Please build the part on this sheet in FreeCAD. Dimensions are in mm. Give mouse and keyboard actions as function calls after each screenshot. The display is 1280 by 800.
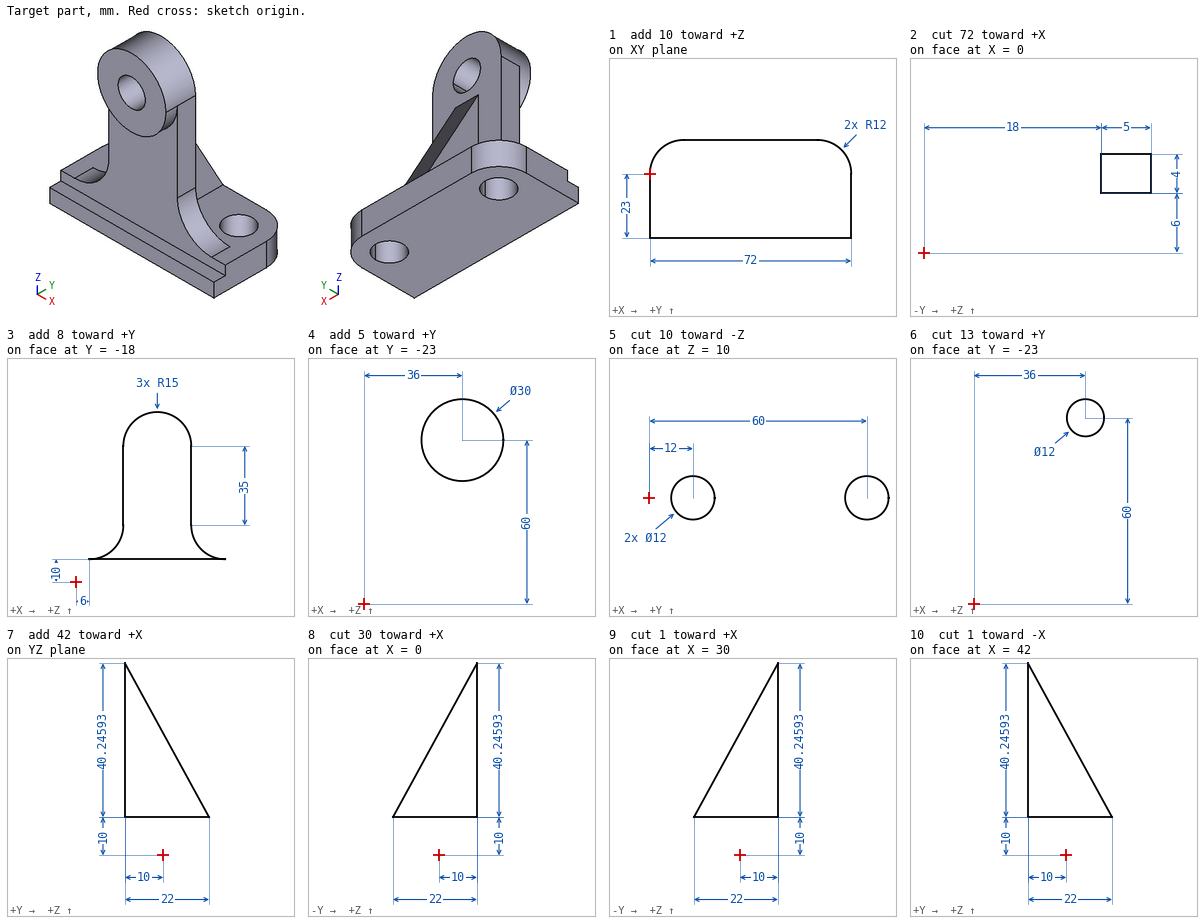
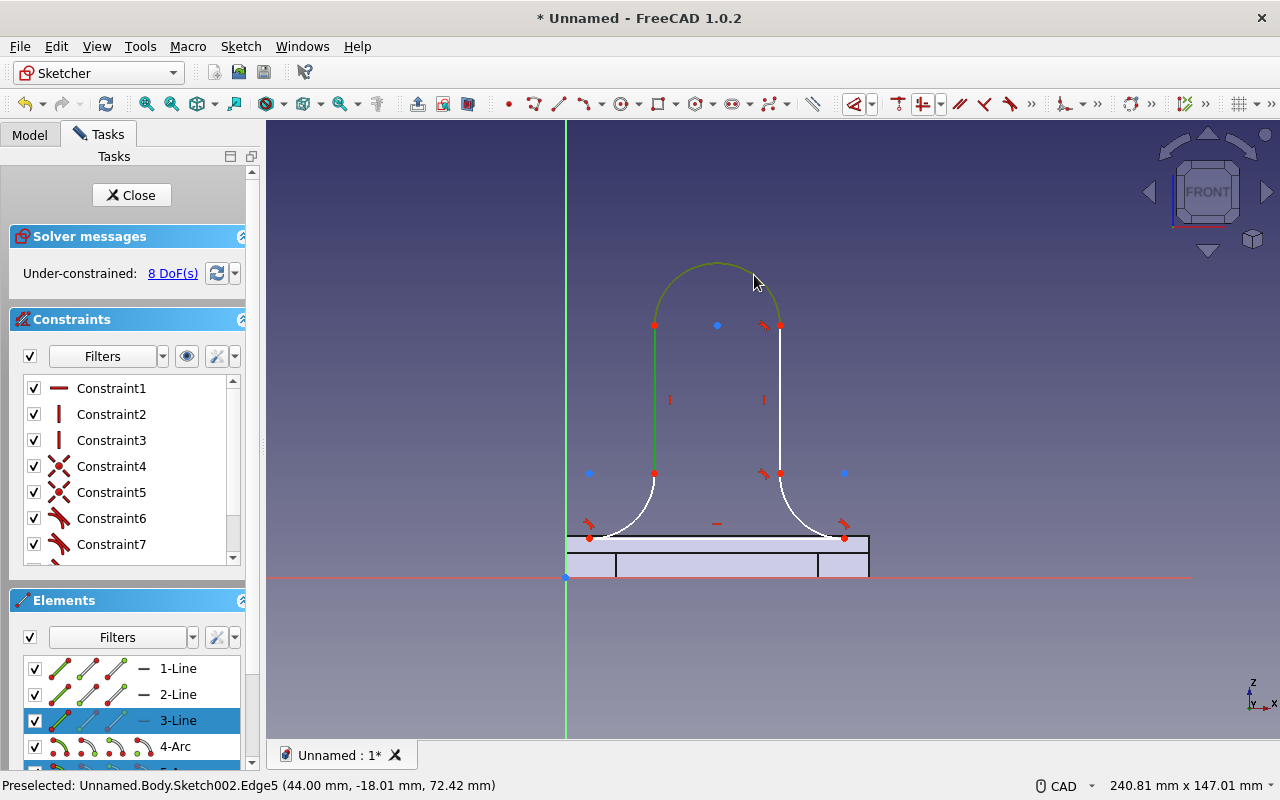
click(1010, 104)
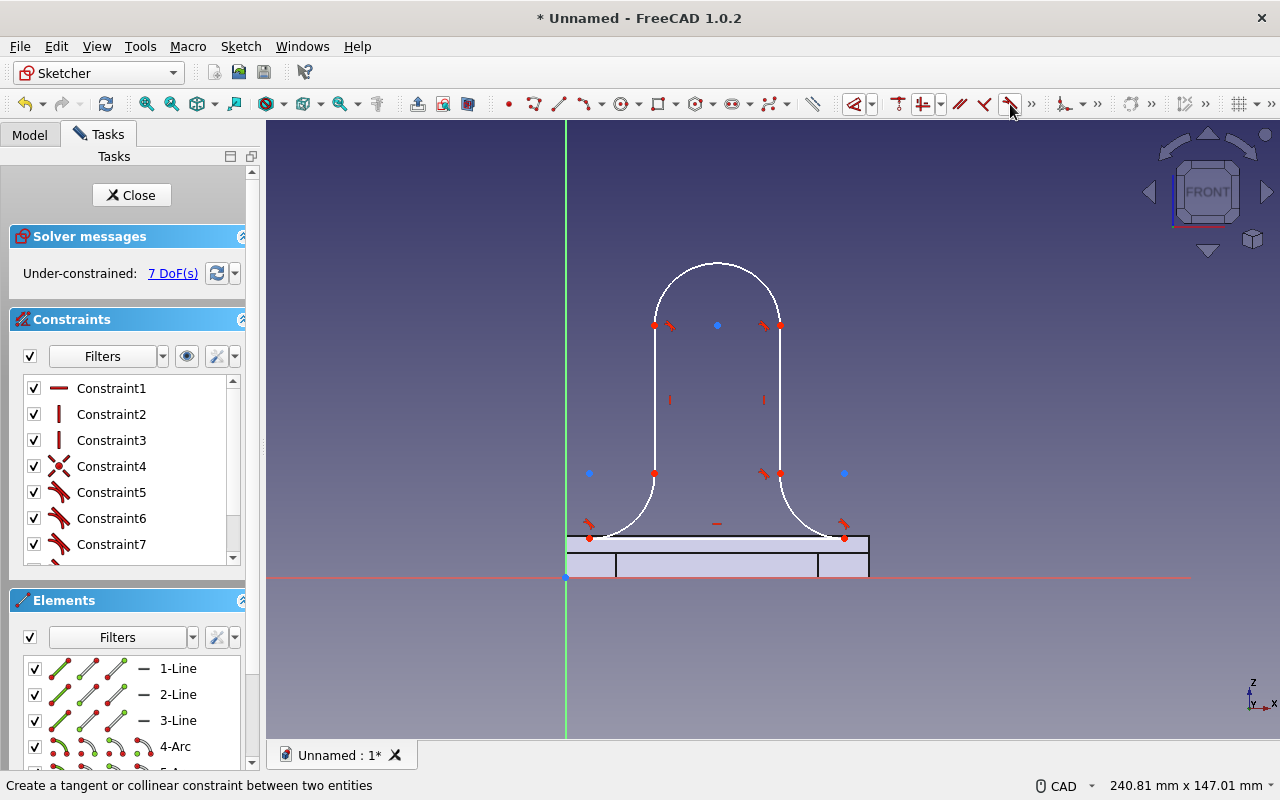
click(655, 370)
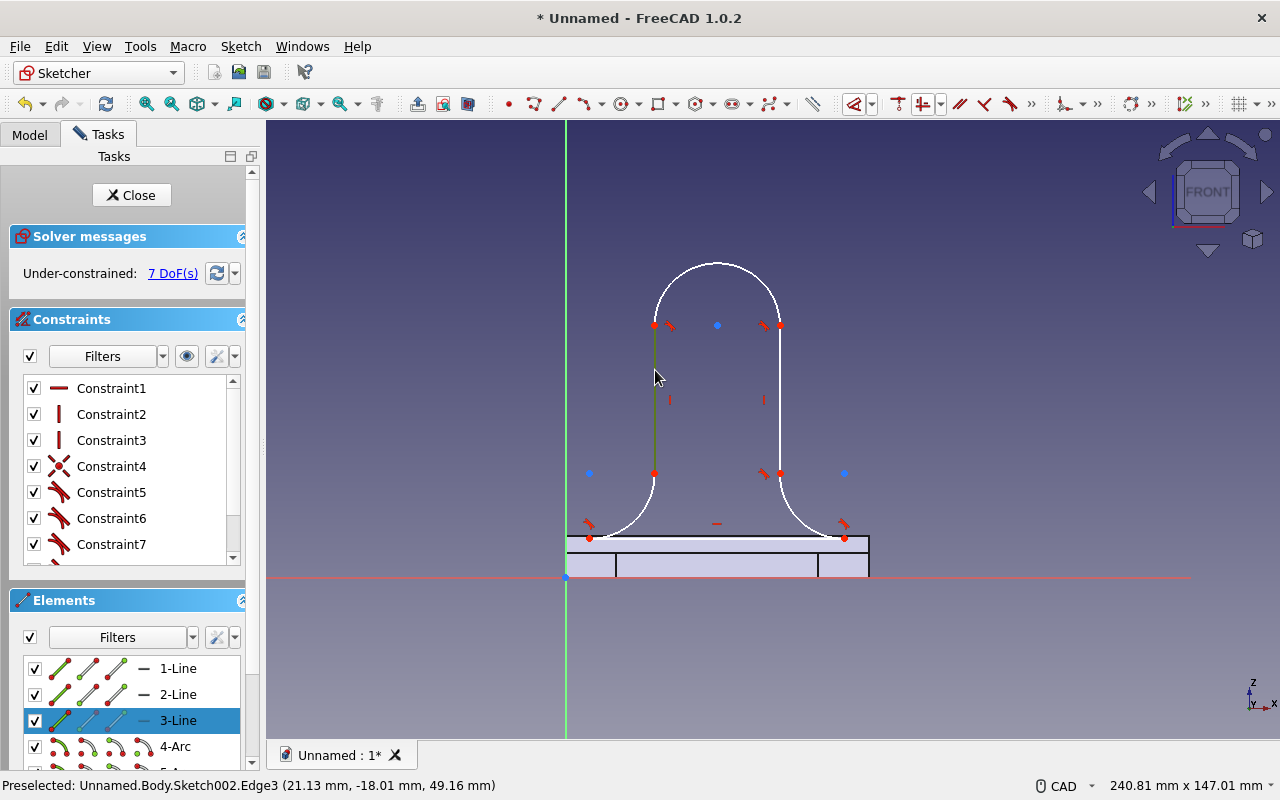
click(647, 503)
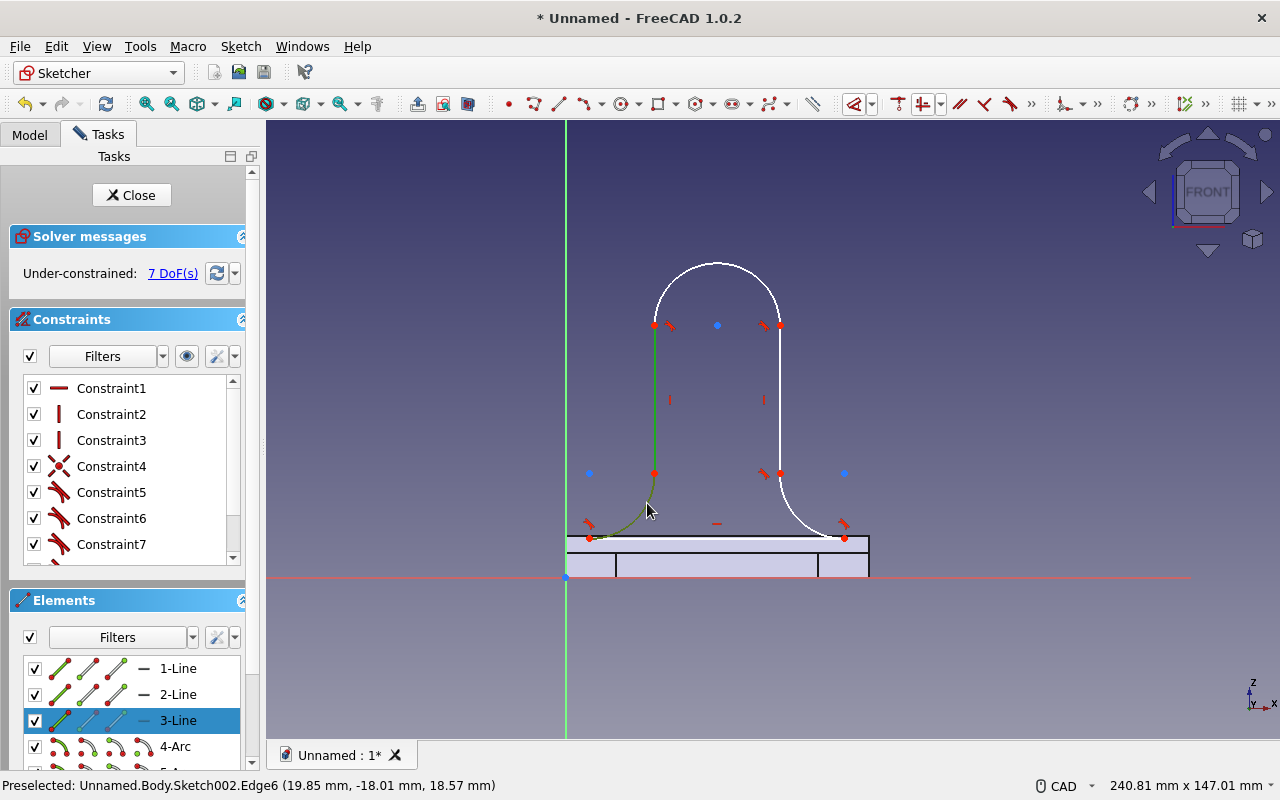
click(1010, 104)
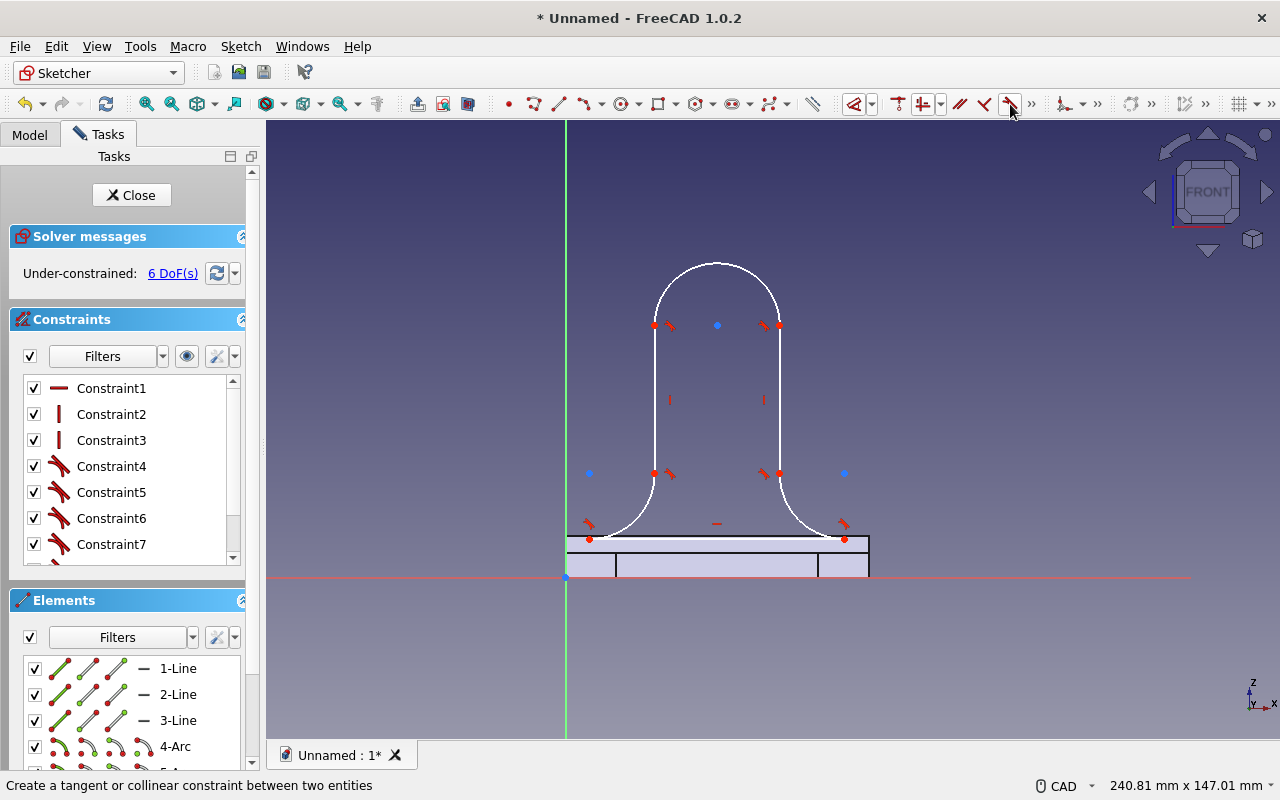
click(787, 504)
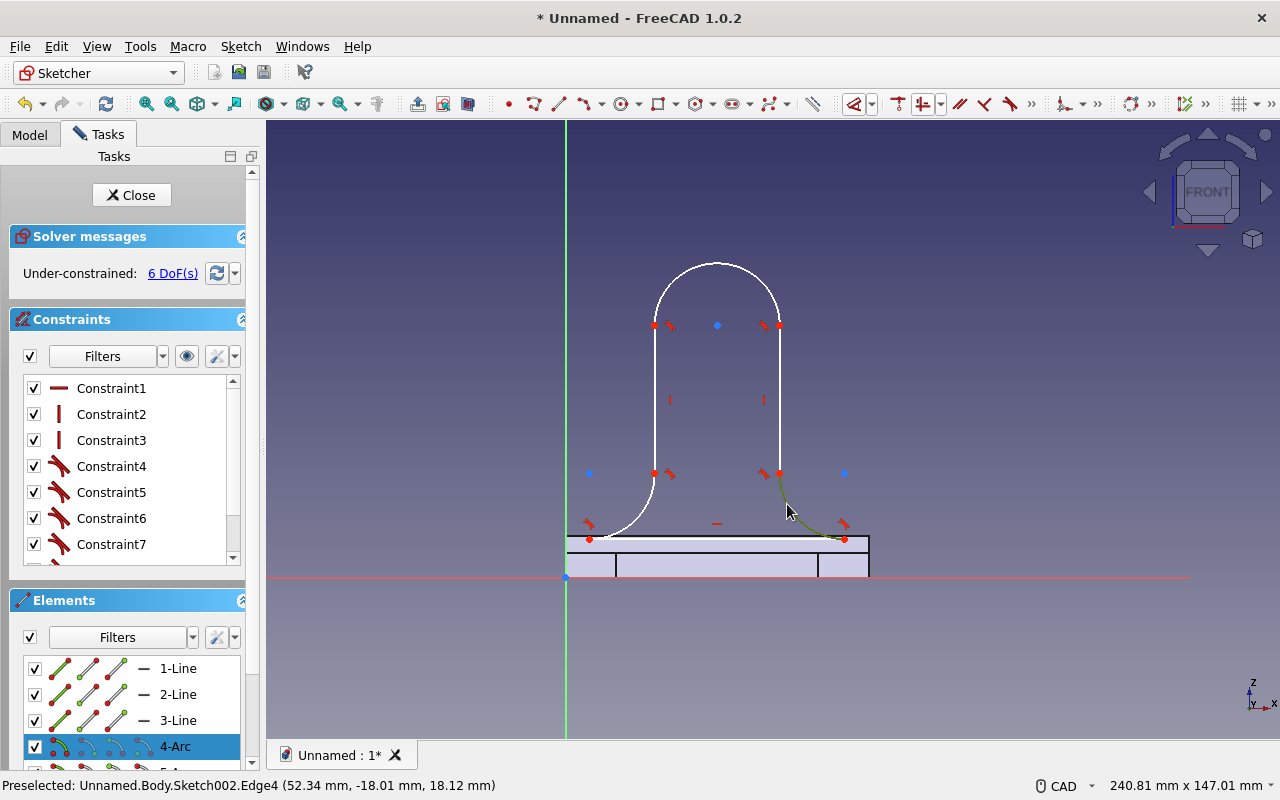
click(754, 275)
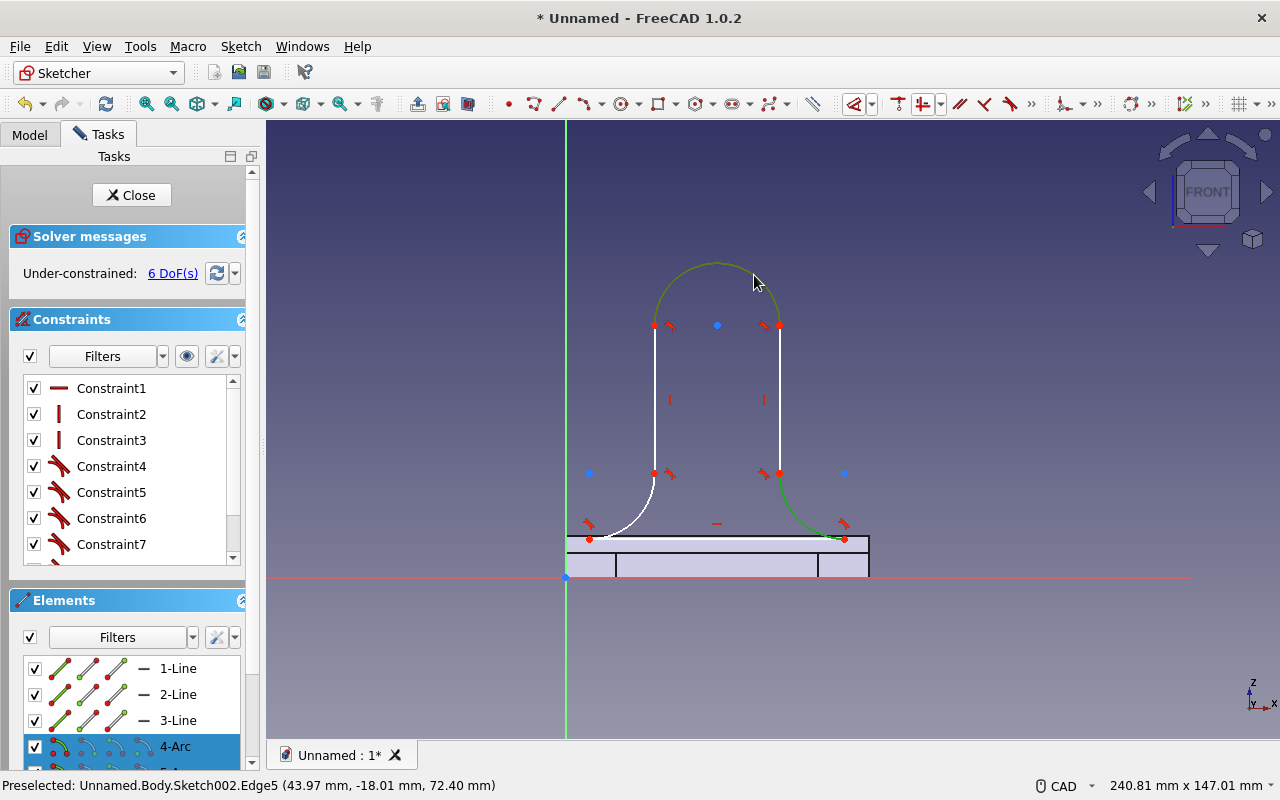
click(648, 504)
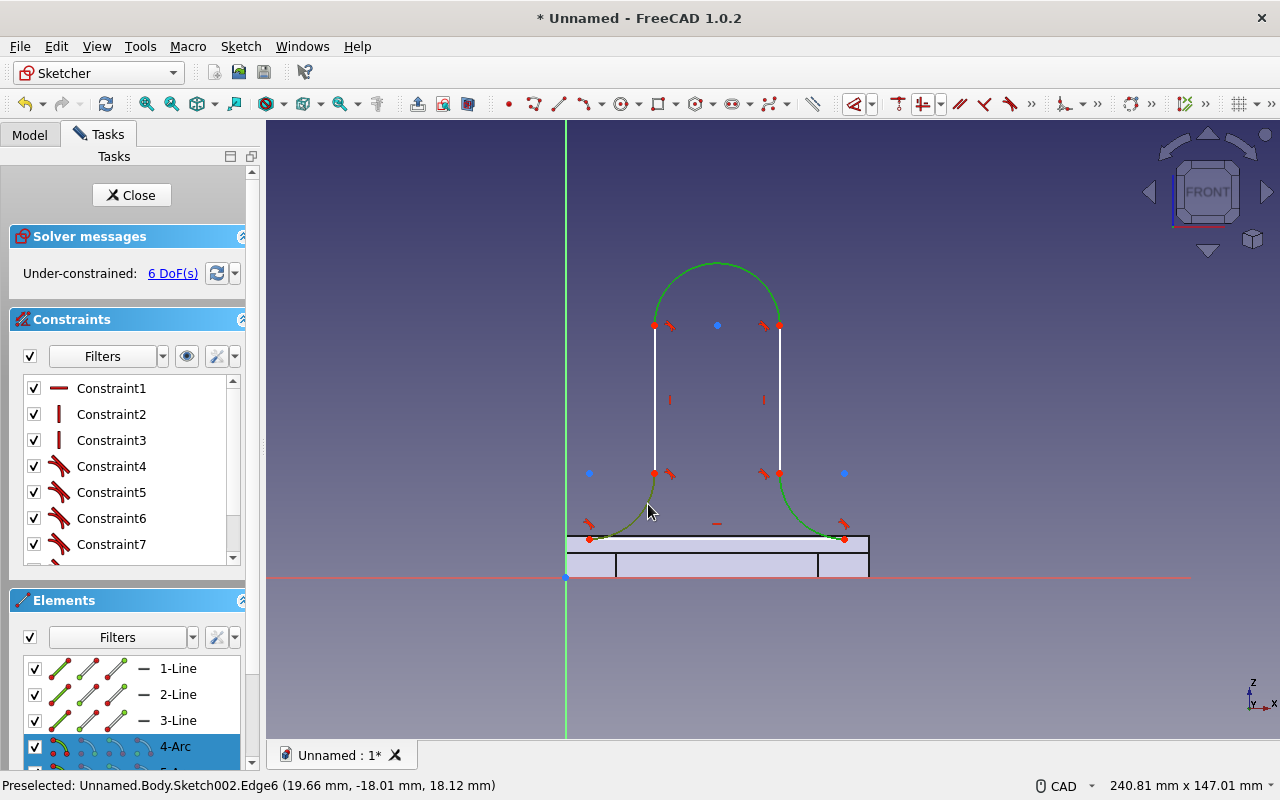
key(e)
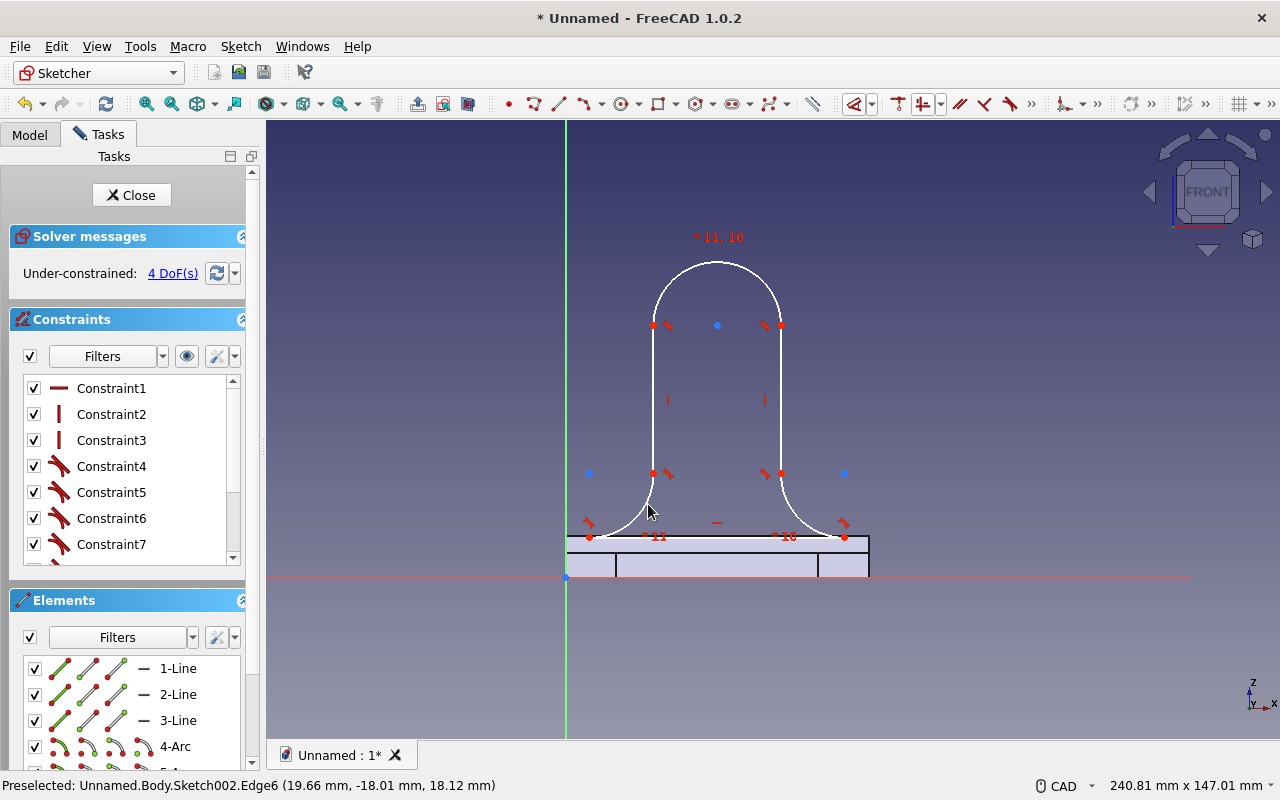
click(788, 503)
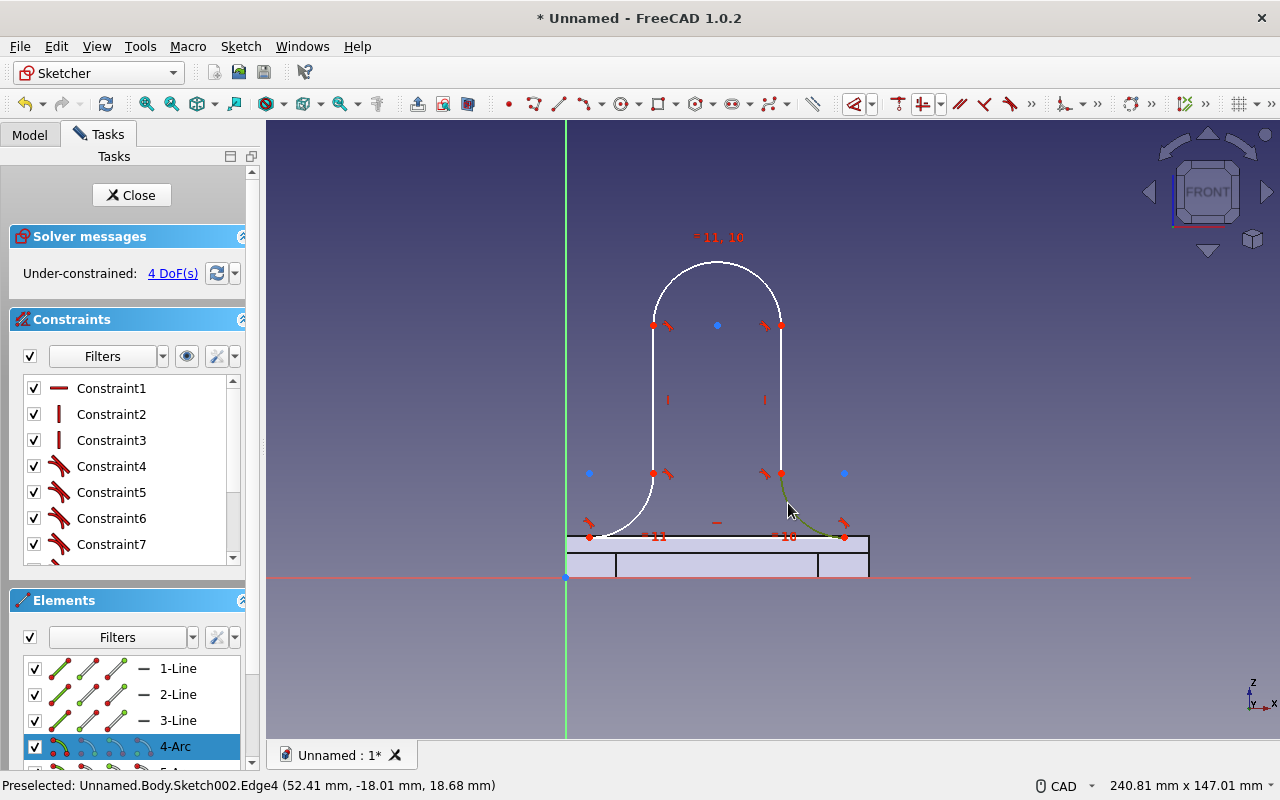
key(k)
key(r)